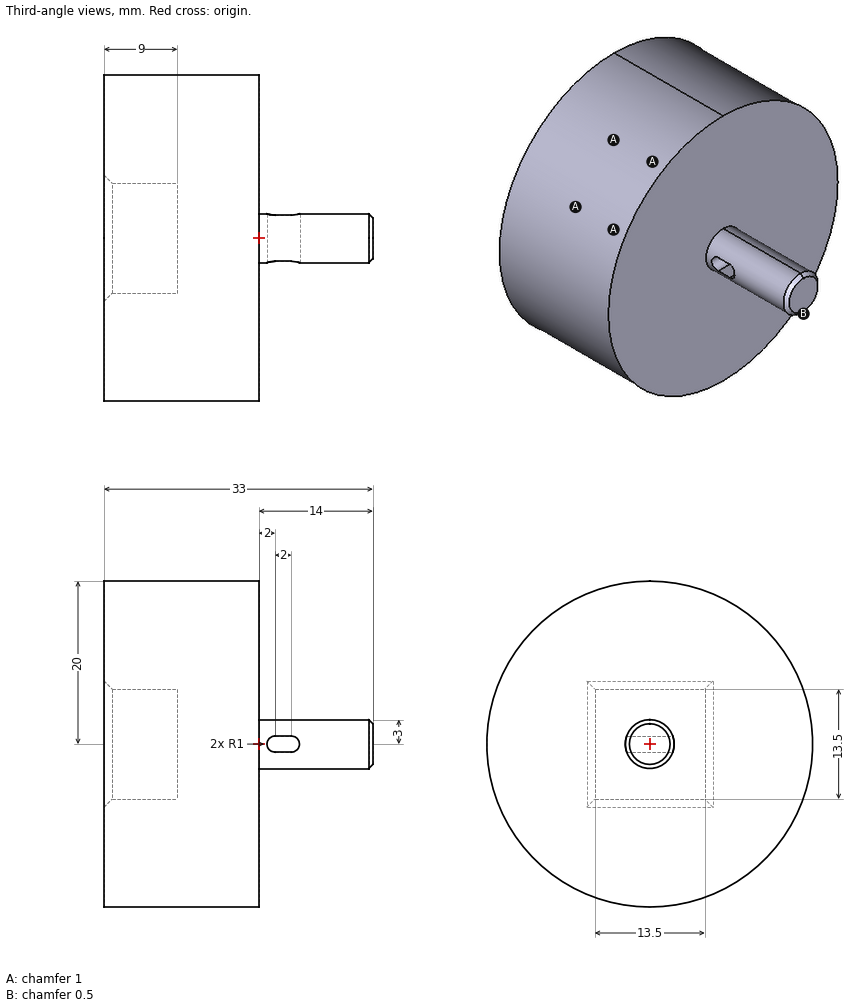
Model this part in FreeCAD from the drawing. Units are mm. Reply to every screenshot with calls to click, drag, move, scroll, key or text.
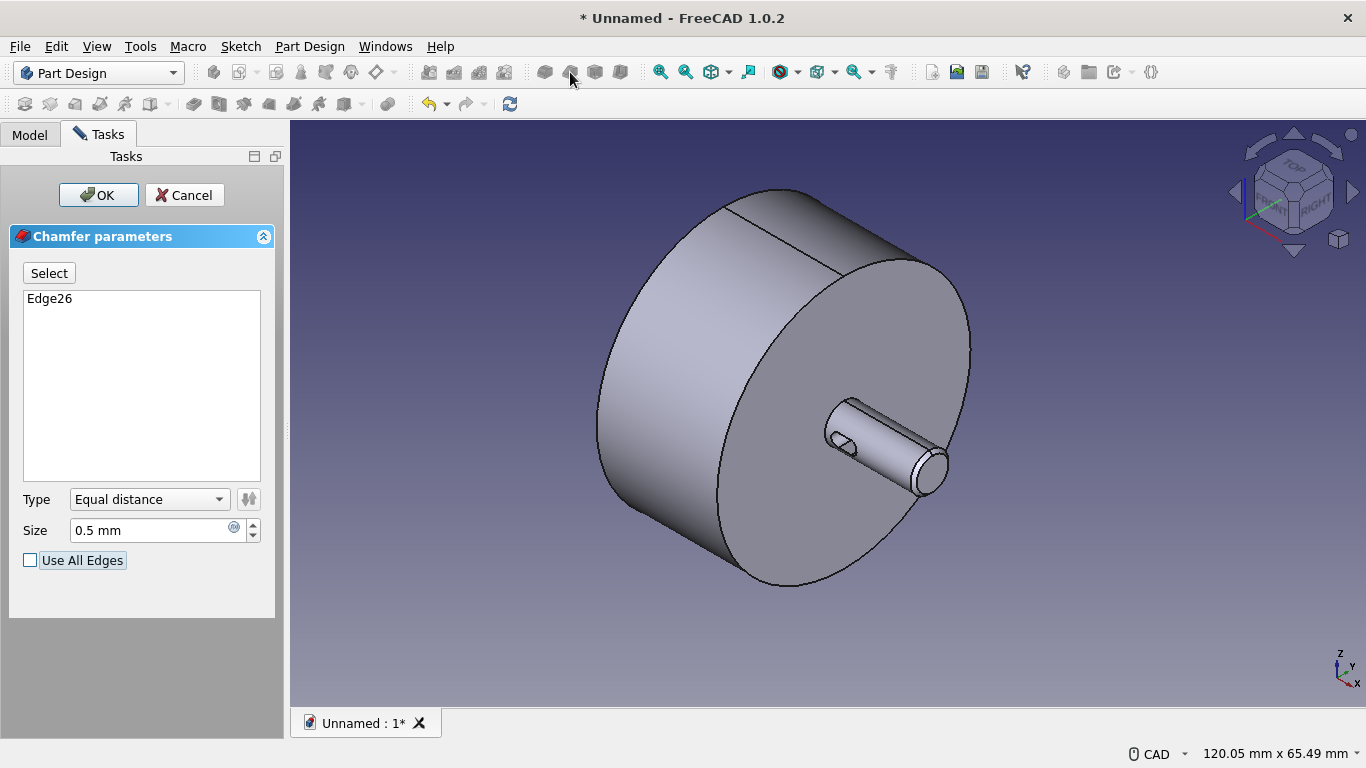
click(99, 195)